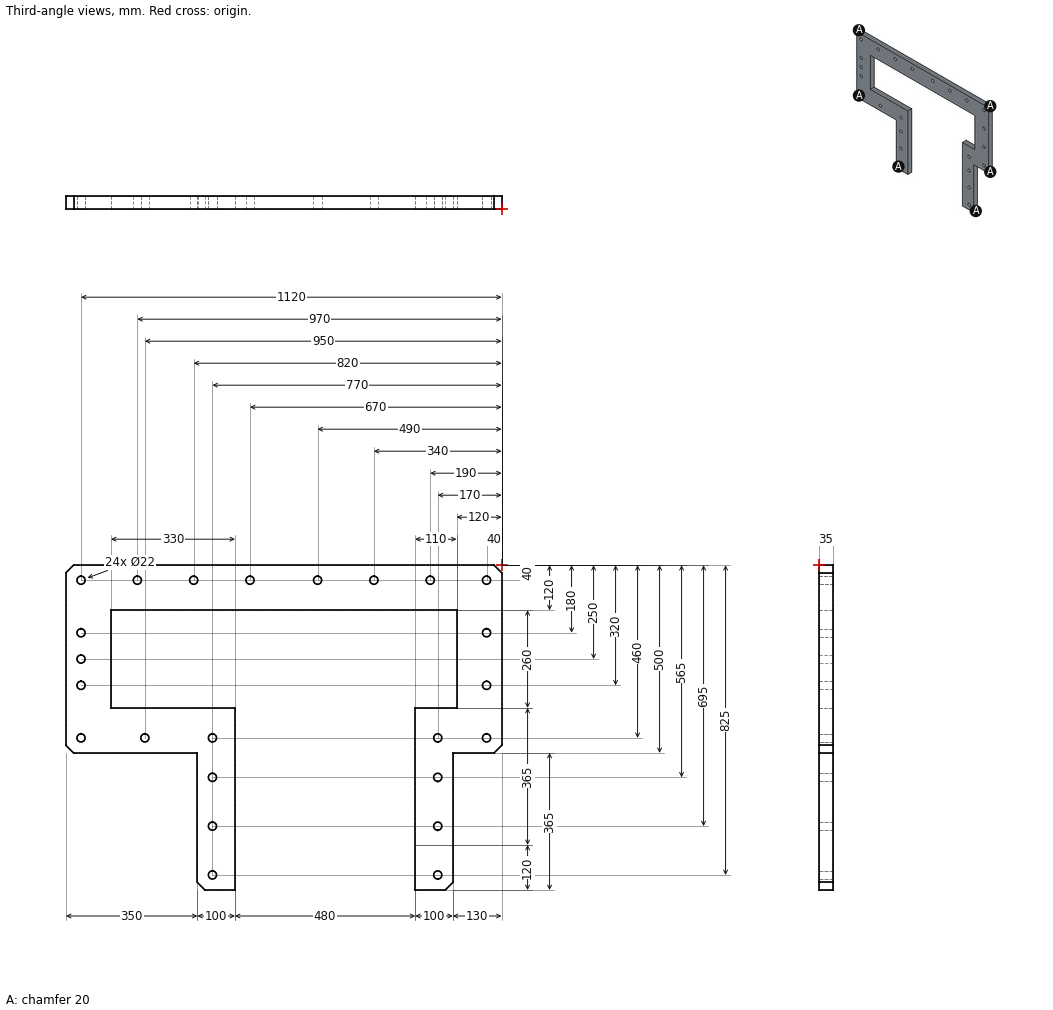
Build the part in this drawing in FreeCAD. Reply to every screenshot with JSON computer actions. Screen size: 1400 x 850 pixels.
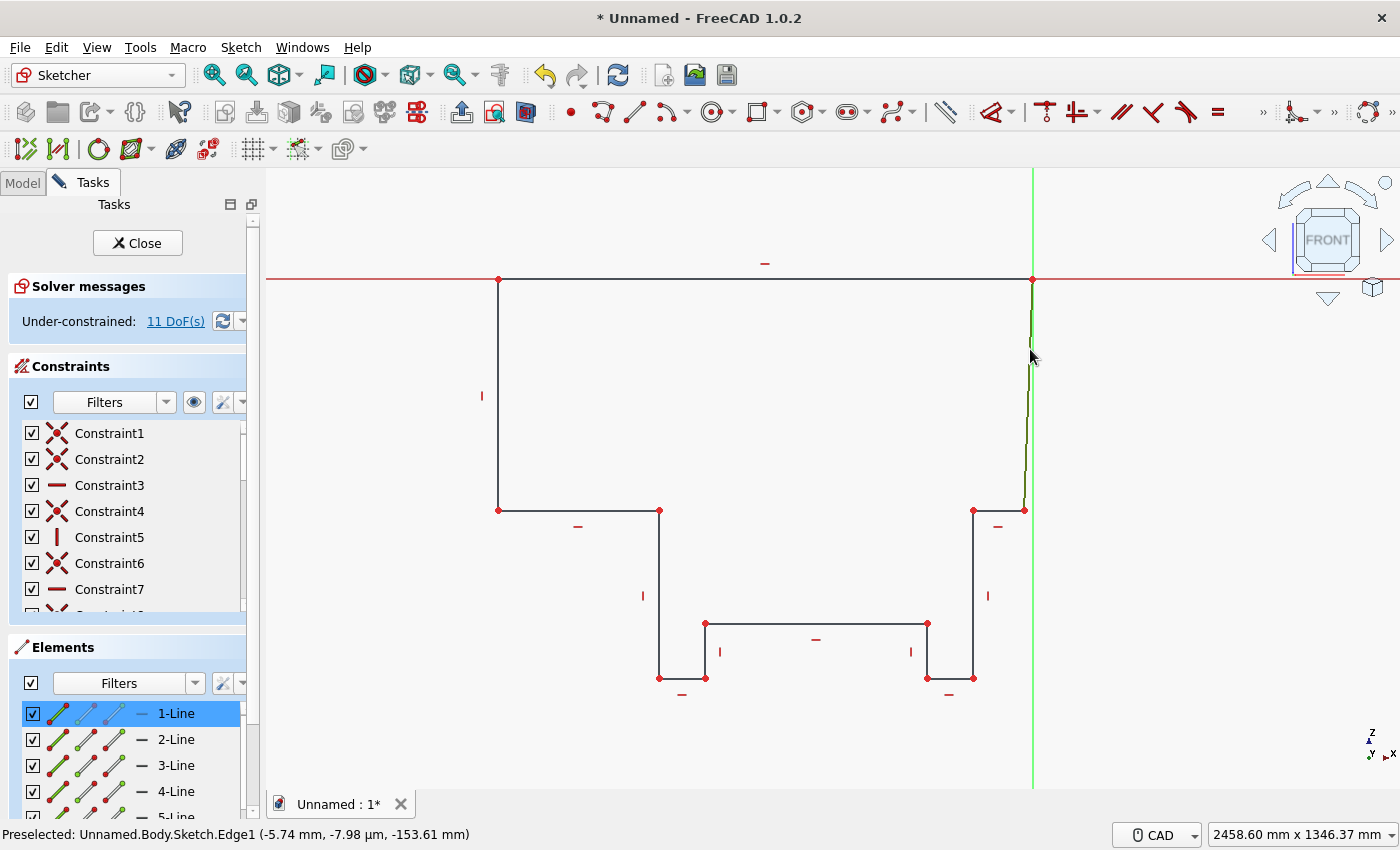
{"action": "left_click", "coordinate": [1100, 112]}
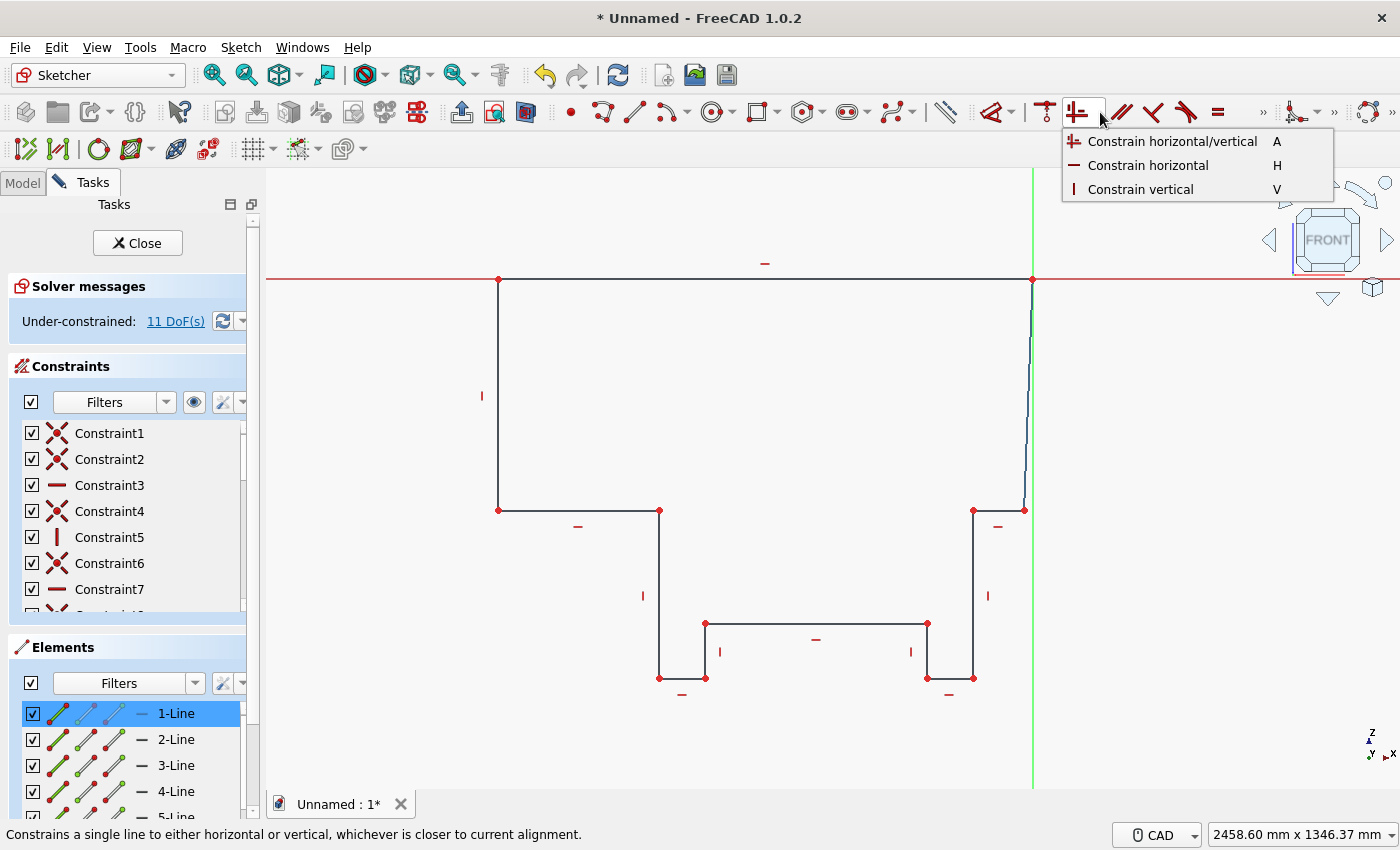
{"action": "left_click", "coordinate": [1198, 189]}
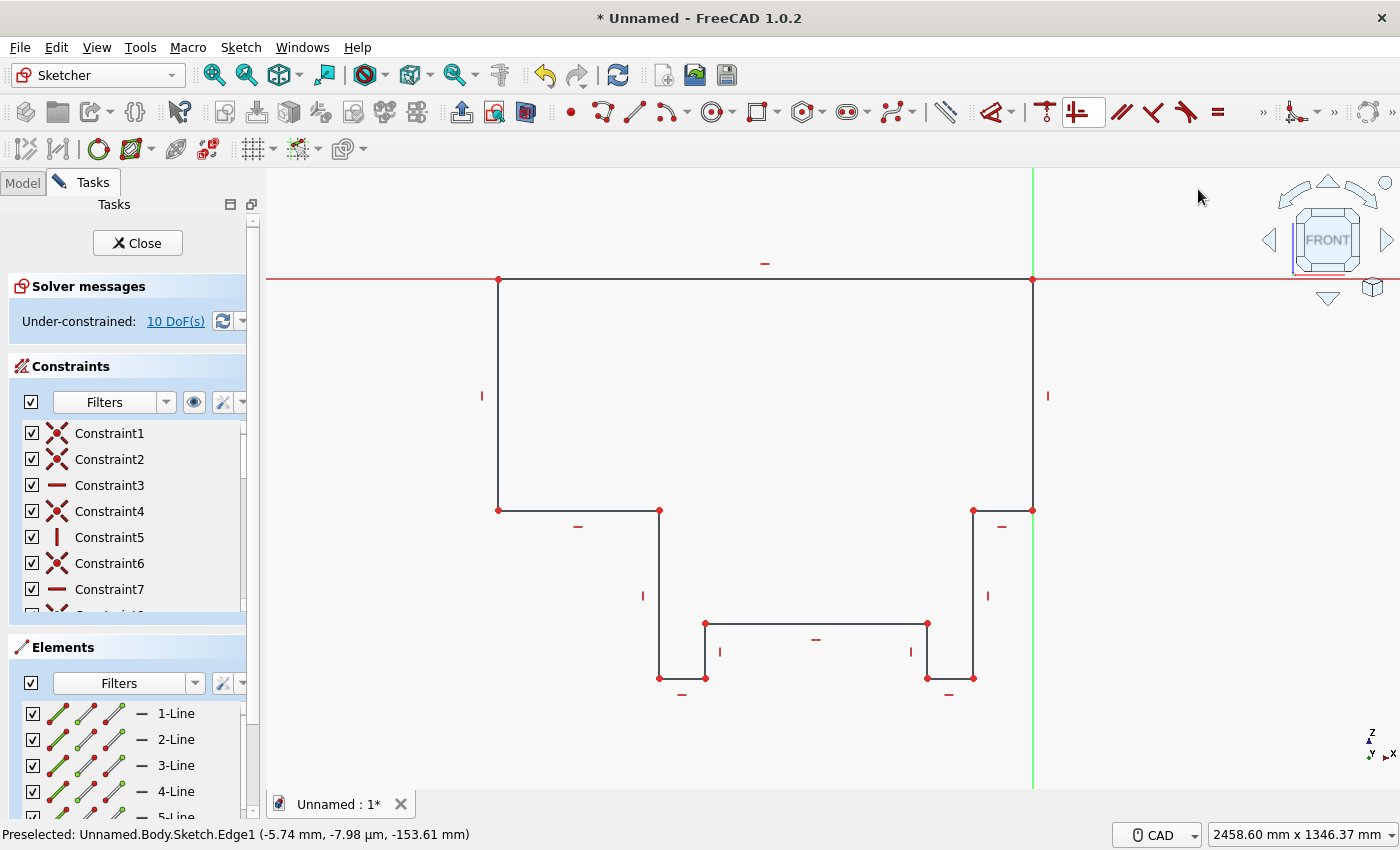
{"action": "left_click", "coordinate": [992, 112]}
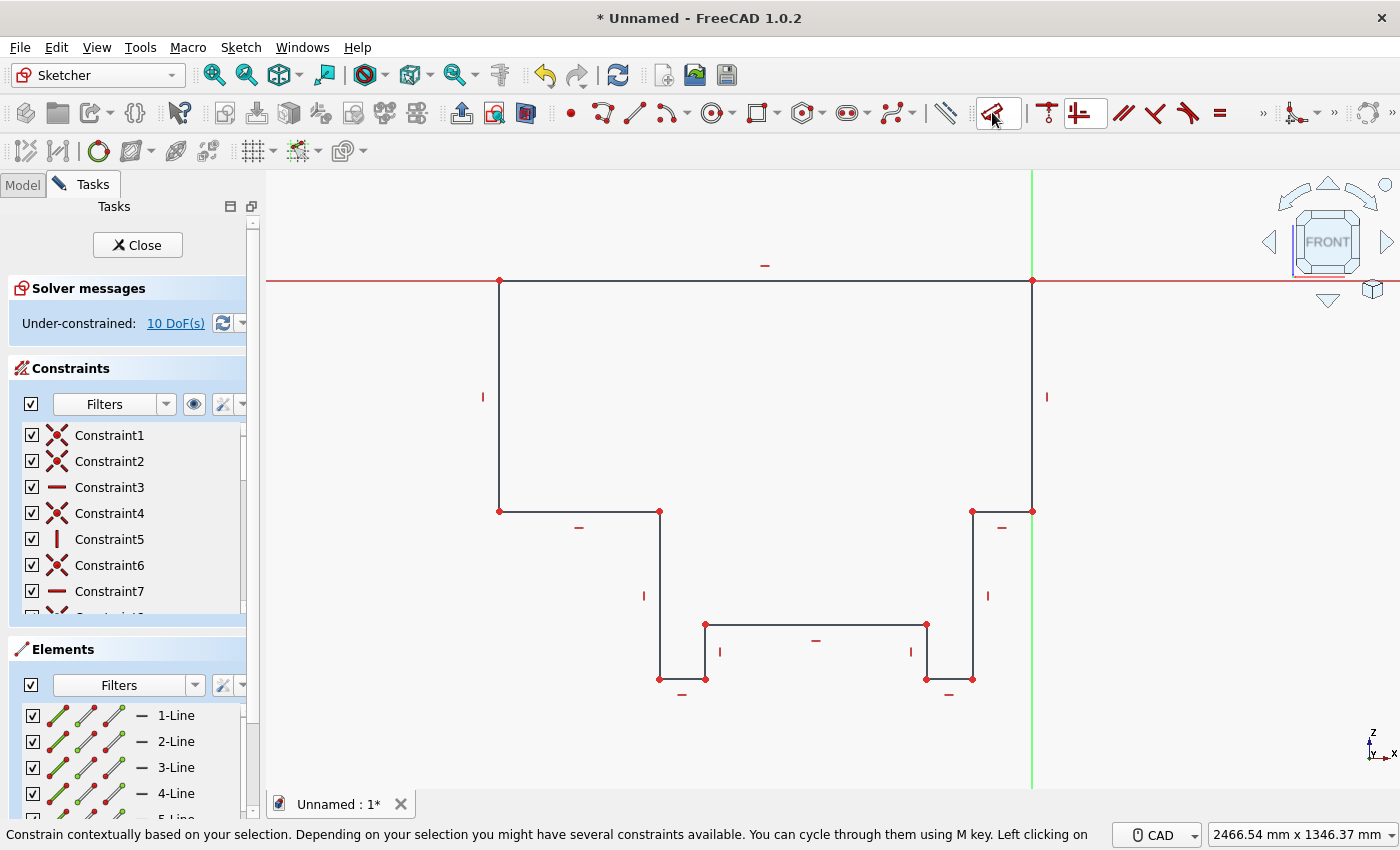
{"action": "left_click", "coordinate": [1032, 350]}
{"action": "left_click", "coordinate": [1066, 396]}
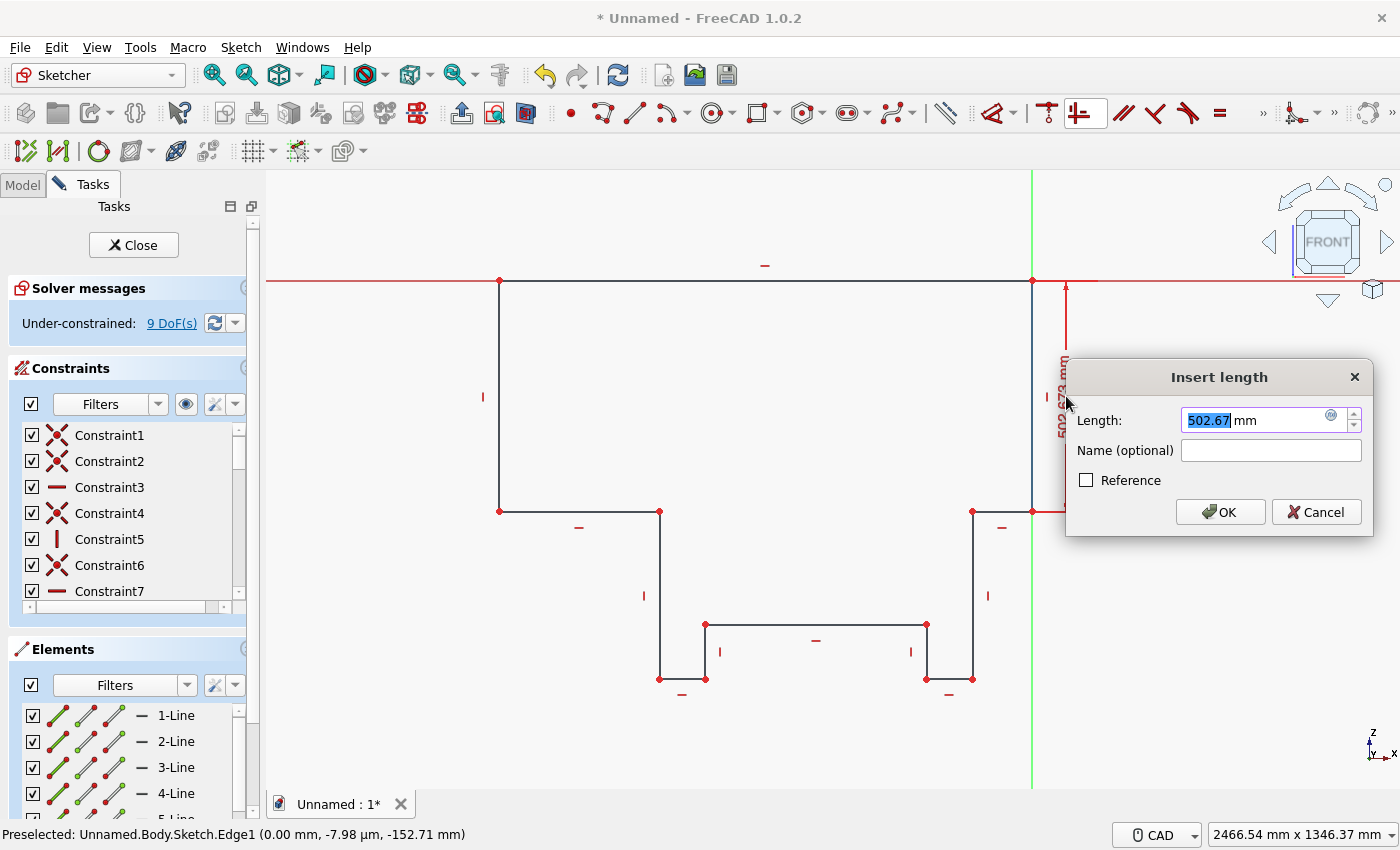
{"action": "type", "text": "500"}
{"action": "key", "text": "Return"}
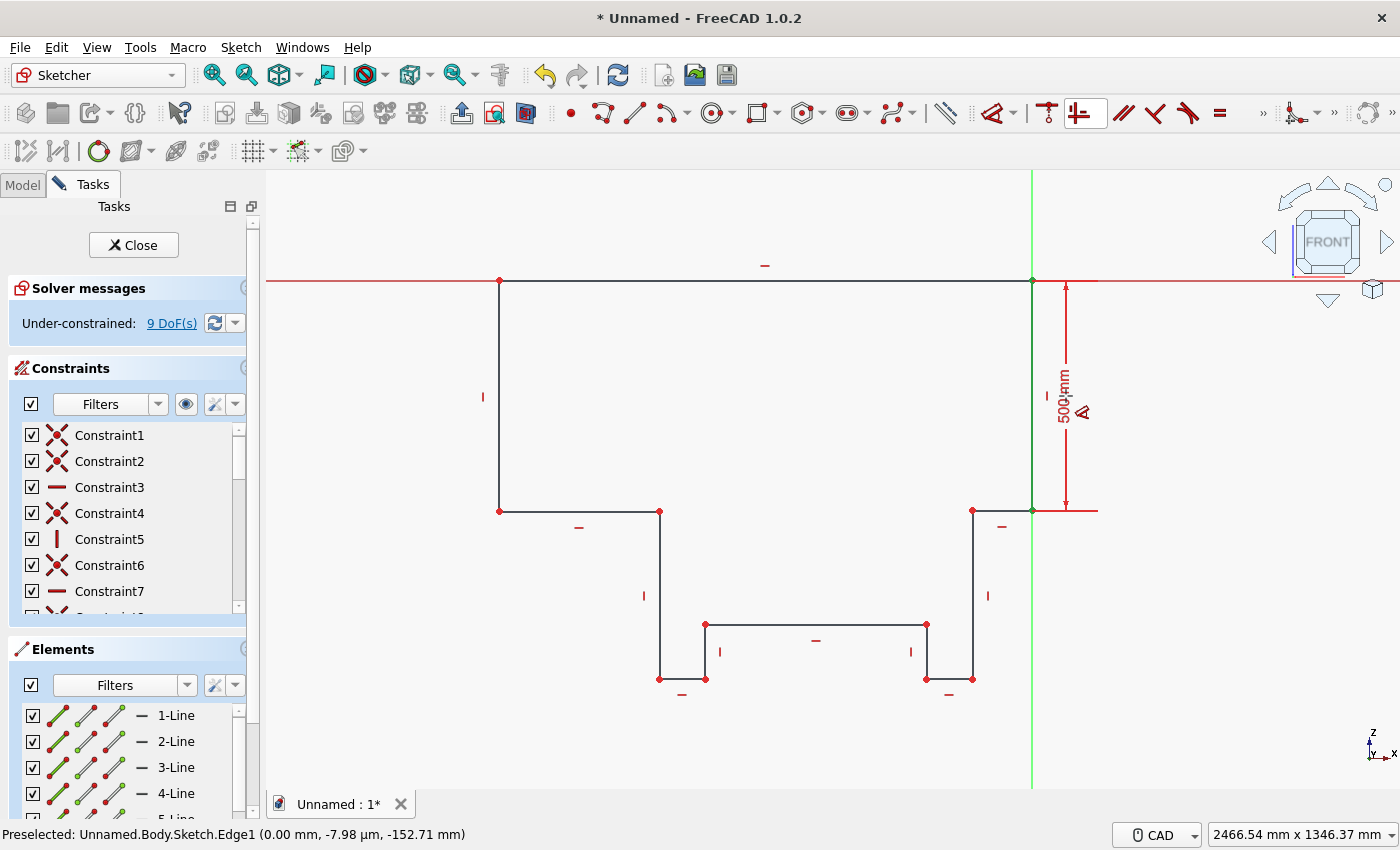
{"action": "left_click", "coordinate": [1014, 511]}
{"action": "left_click", "coordinate": [1002, 545]}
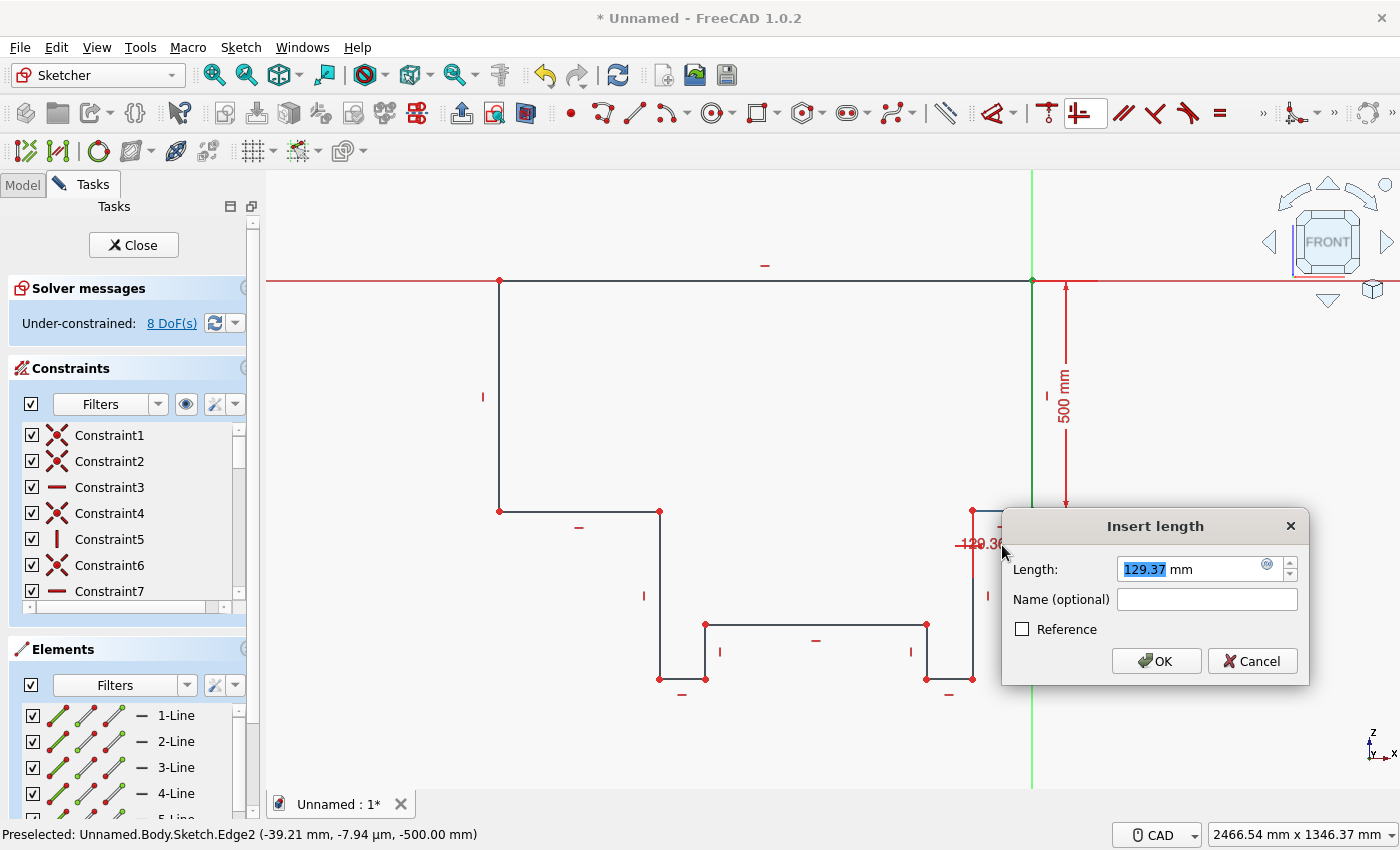
{"action": "type", "text": "130"}
{"action": "key", "text": "Return"}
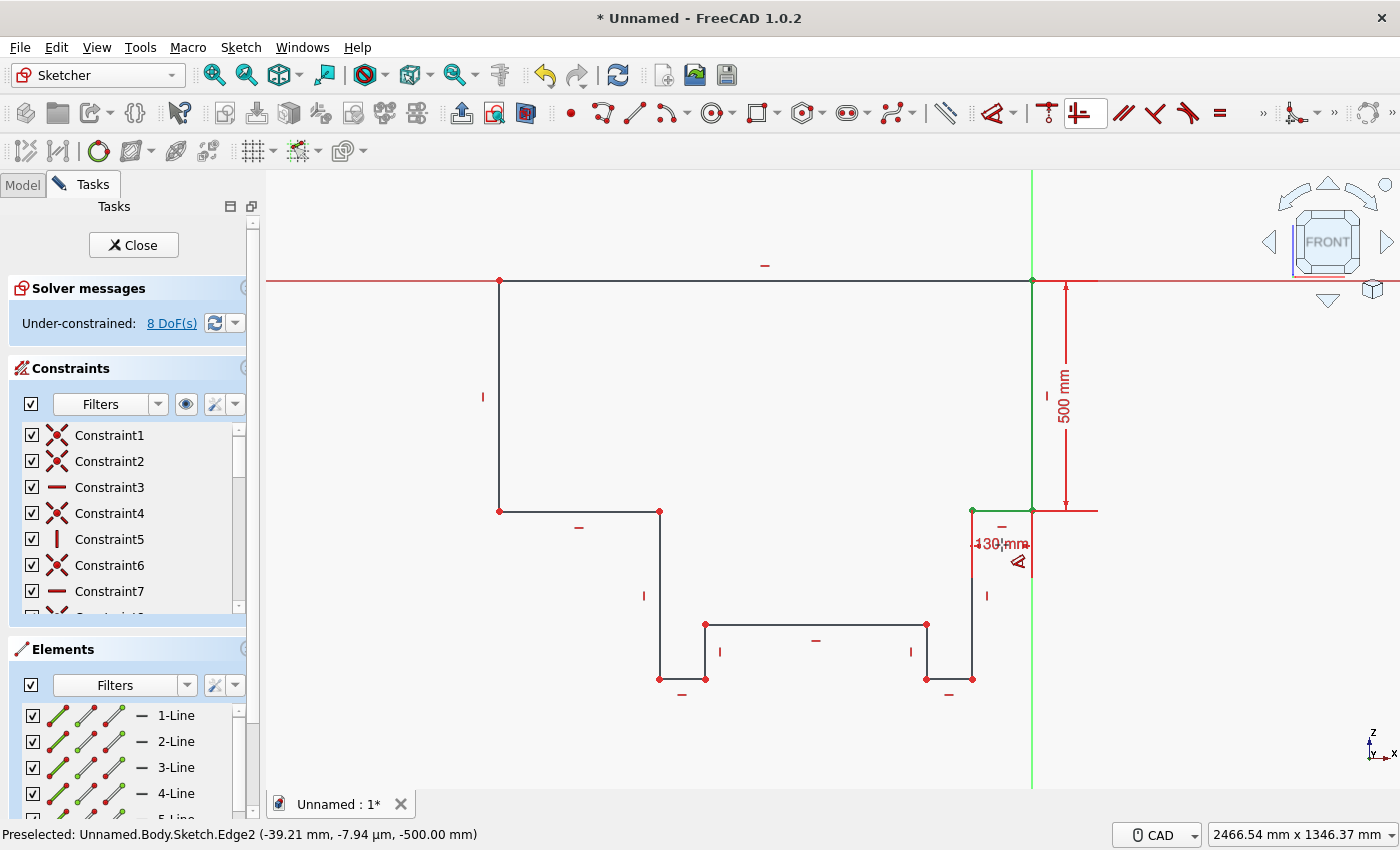
{"action": "left_click", "coordinate": [972, 561]}
{"action": "left_click", "coordinate": [1006, 595]}